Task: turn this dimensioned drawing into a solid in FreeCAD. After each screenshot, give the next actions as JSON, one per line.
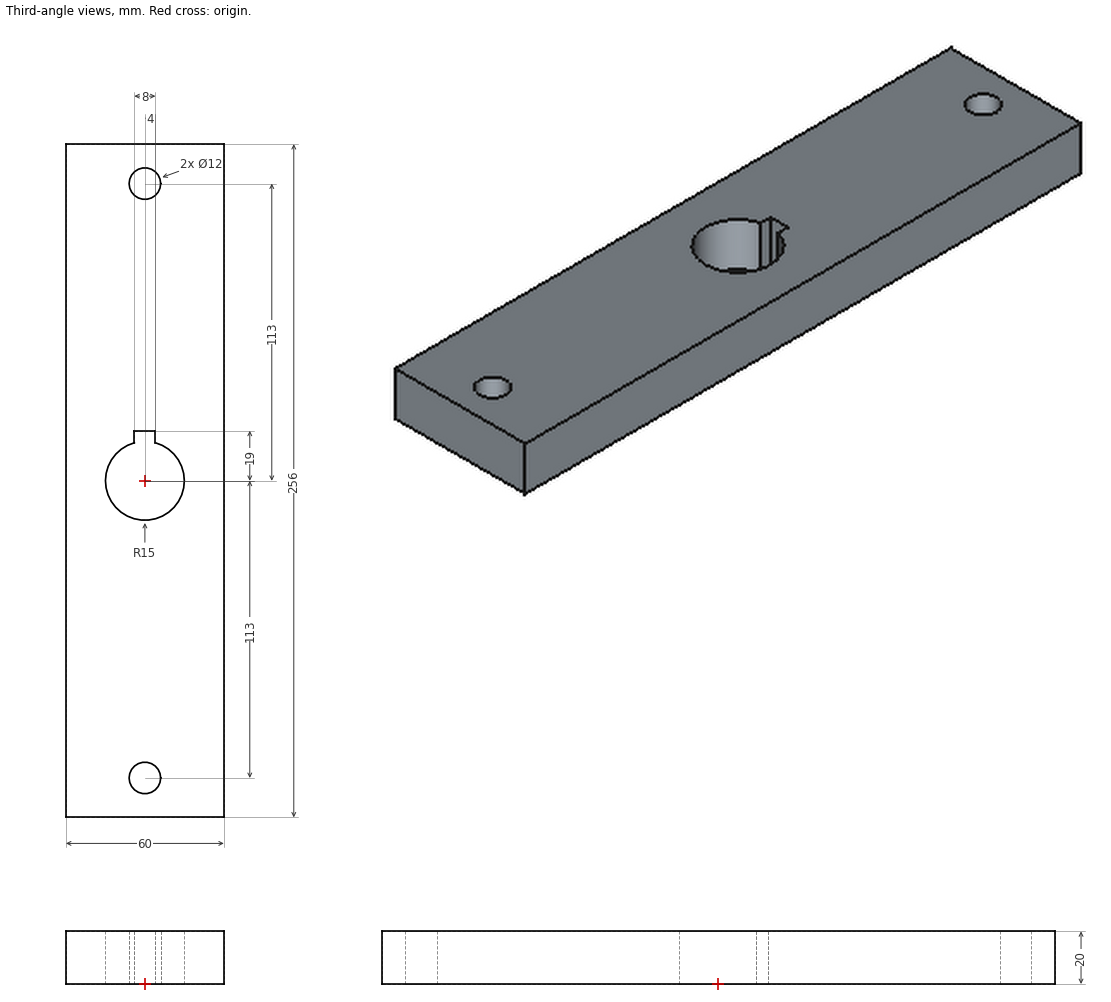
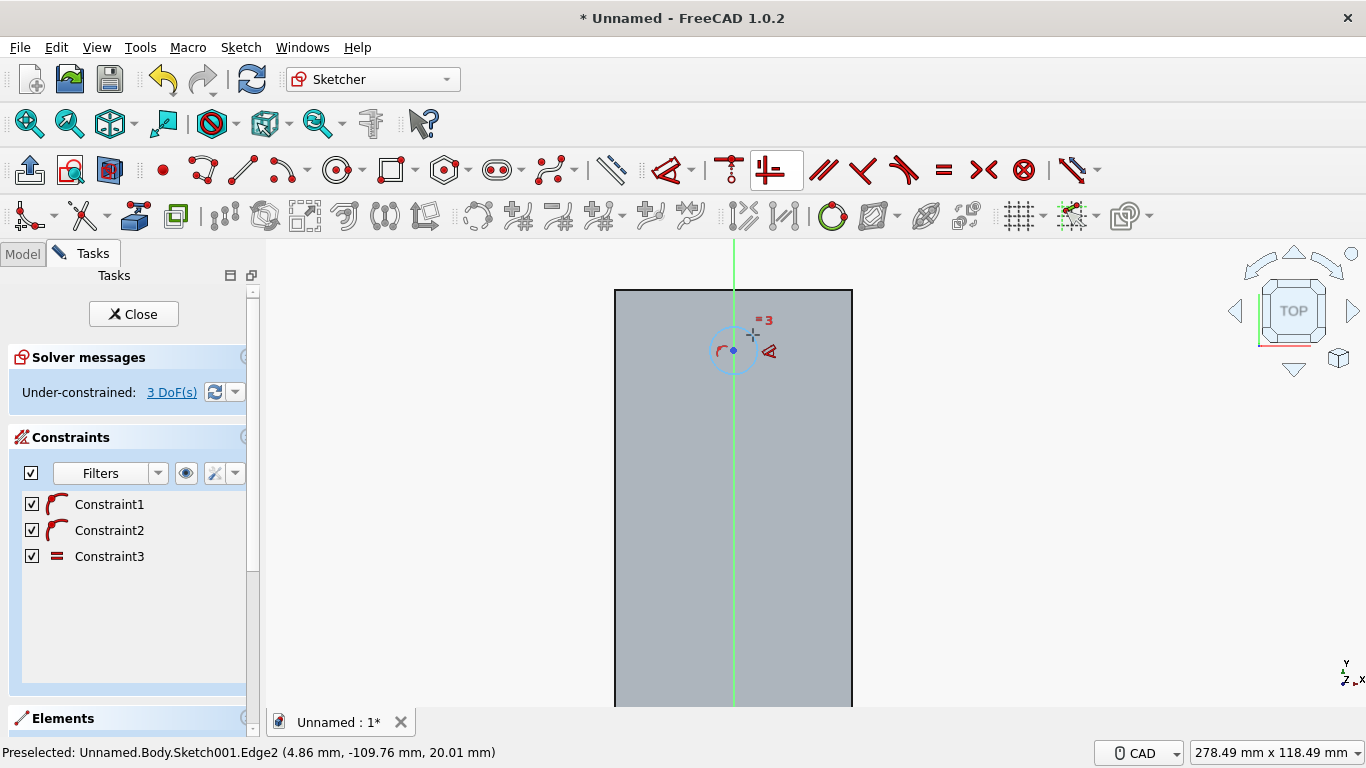
{"action": "left_click", "coordinate": [751, 334]}
{"action": "left_click", "coordinate": [774, 312]}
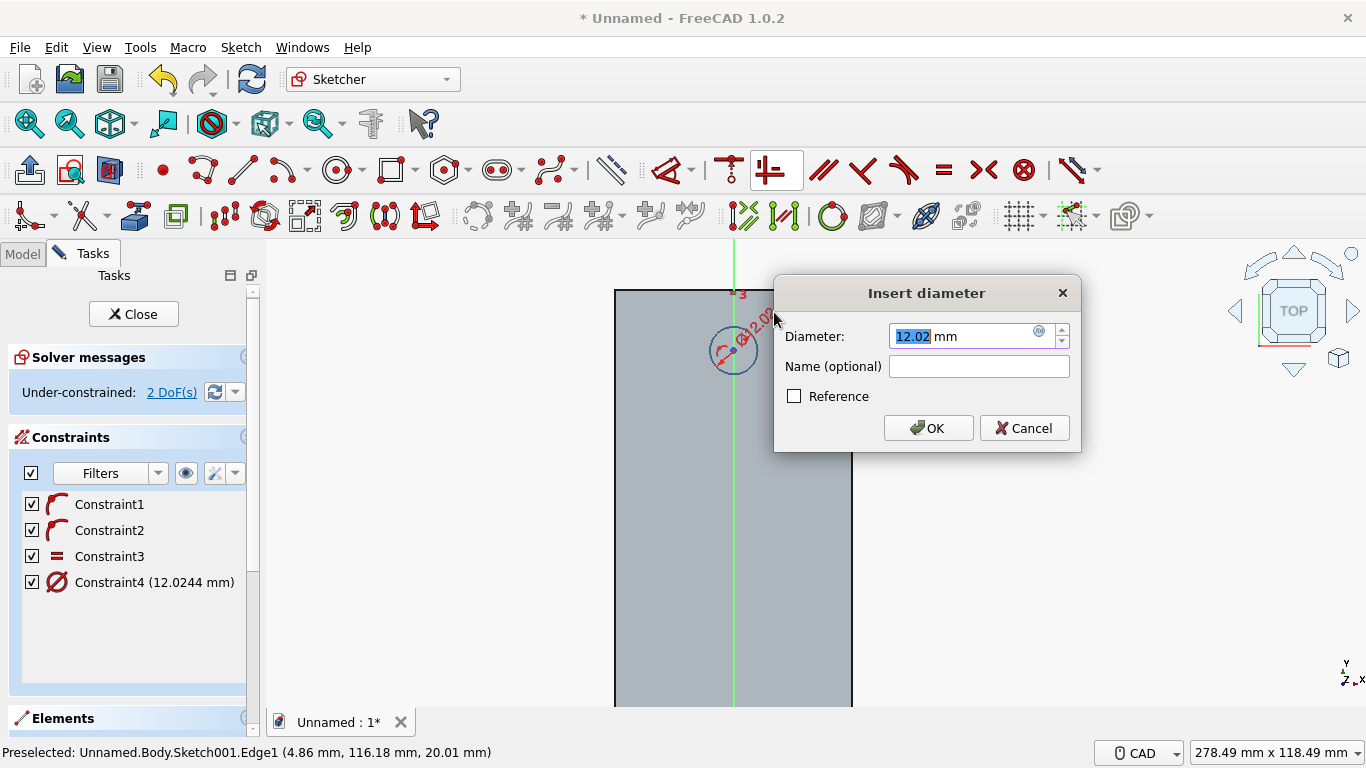
{"action": "type", "text": "12"}
{"action": "key", "text": "Return"}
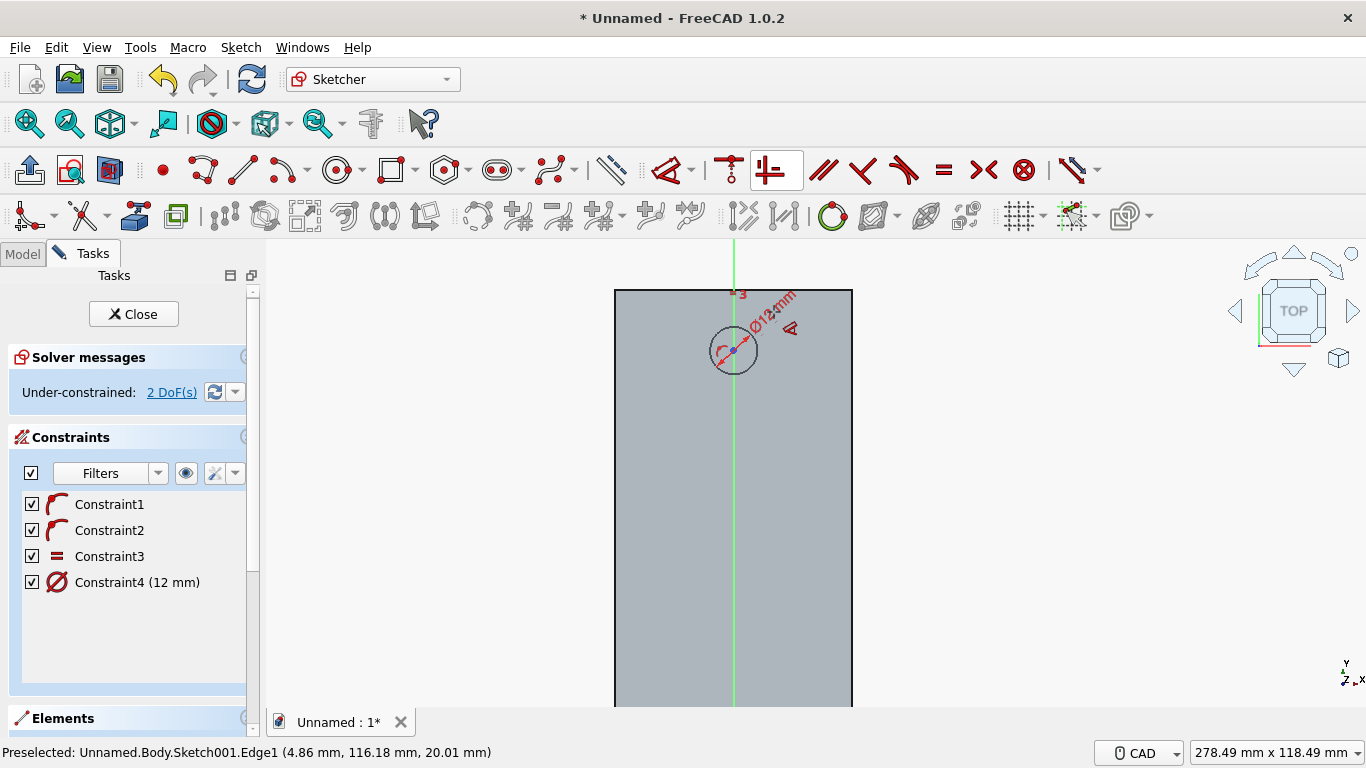
{"action": "left_click", "coordinate": [734, 351]}
{"action": "left_click", "coordinate": [768, 515]}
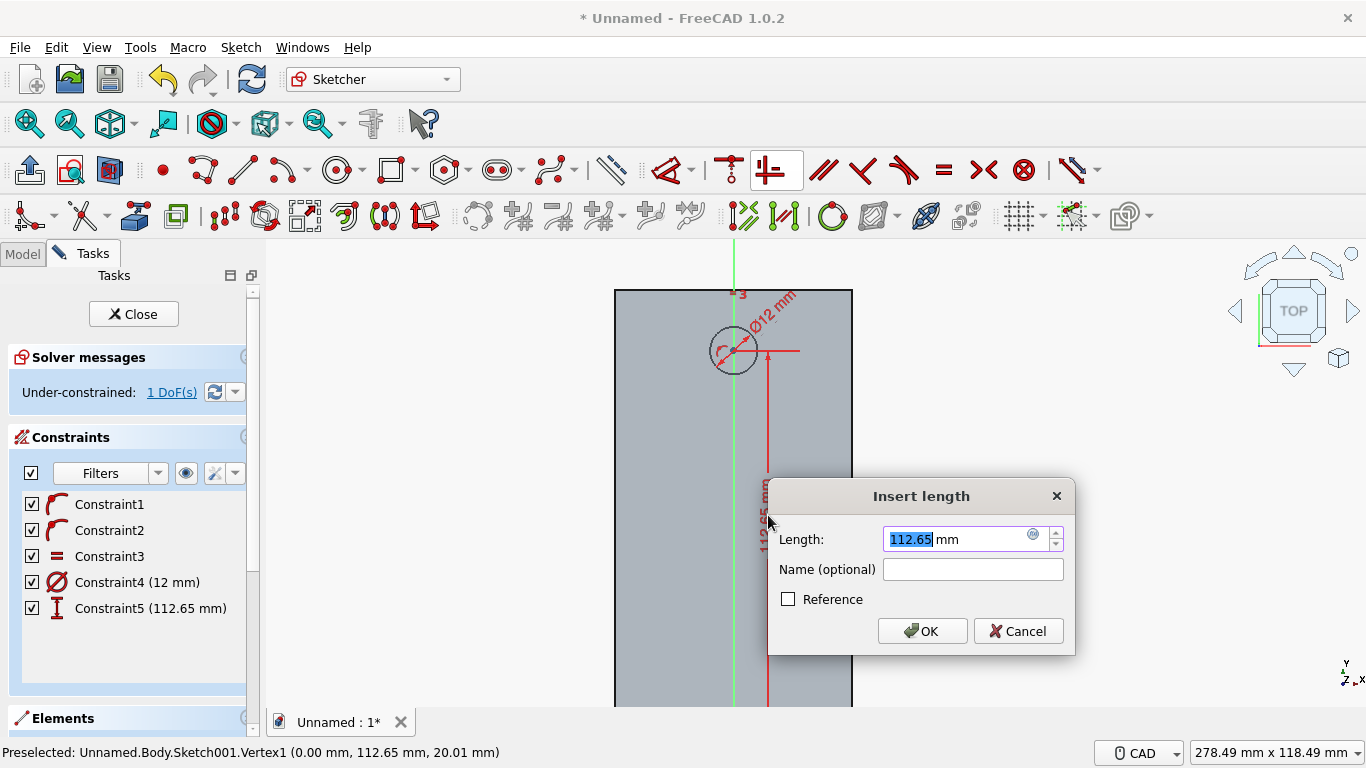
{"action": "type", "text": "113"}
{"action": "key", "text": "Return"}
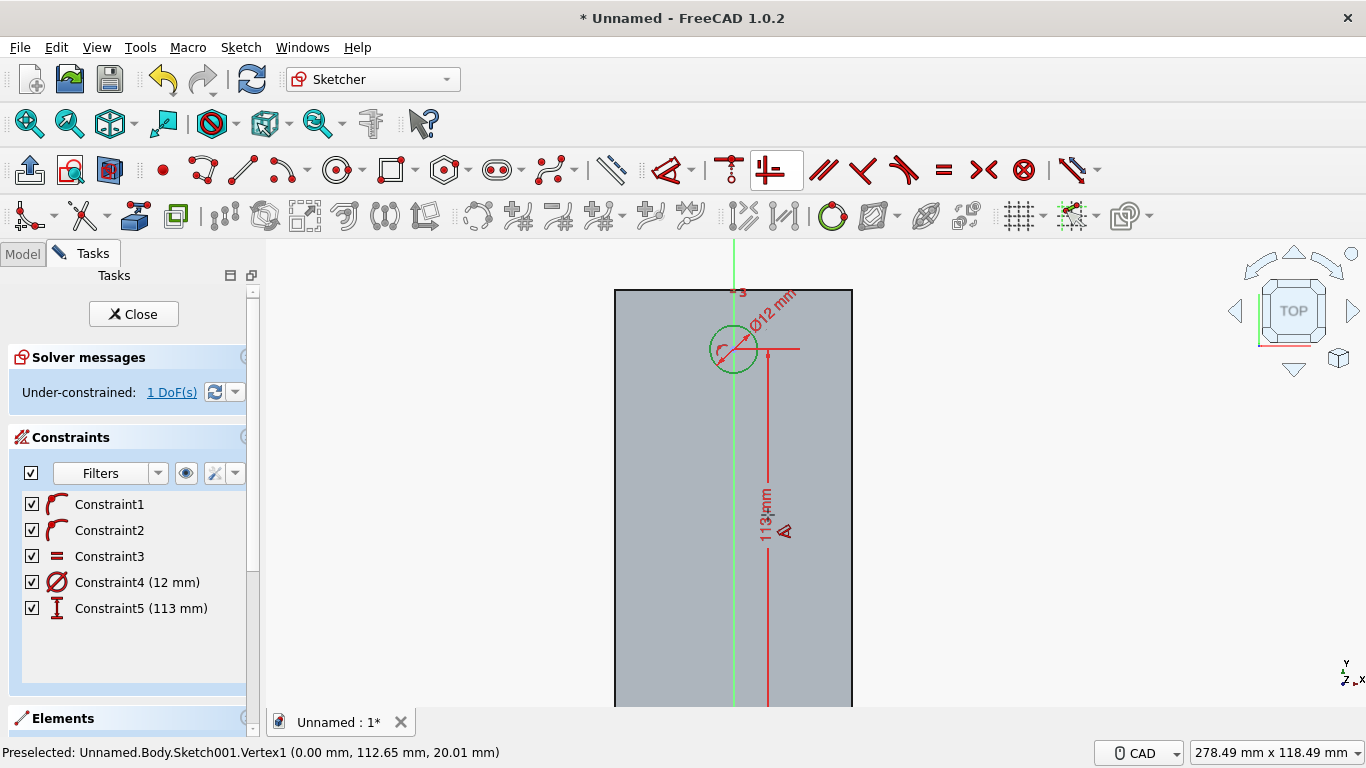
{"action": "scroll", "coordinate": [753, 334], "scroll_direction": "down", "scroll_amount": 6}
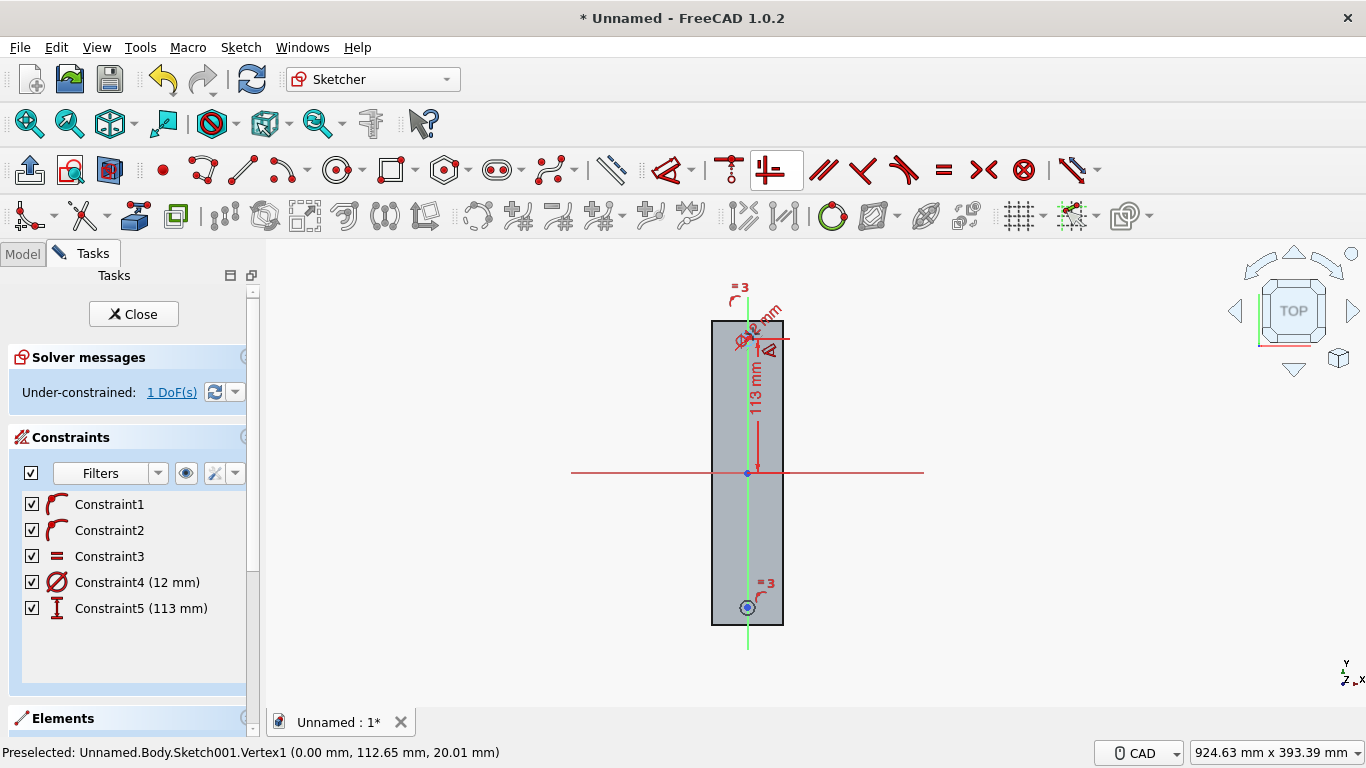
{"action": "left_click", "coordinate": [748, 608]}
{"action": "left_click", "coordinate": [782, 541]}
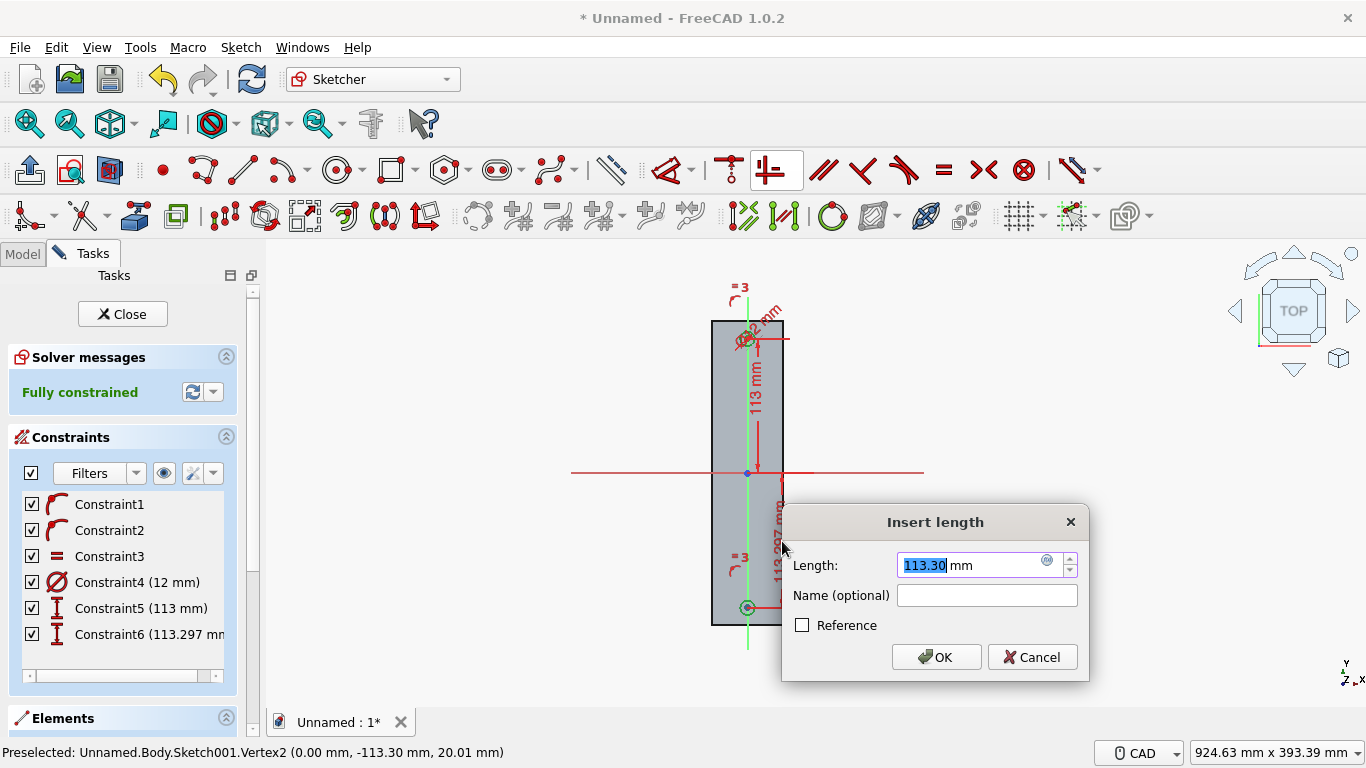
{"action": "type", "text": "113"}
{"action": "key", "text": "Return"}
{"action": "key", "text": "Escape"}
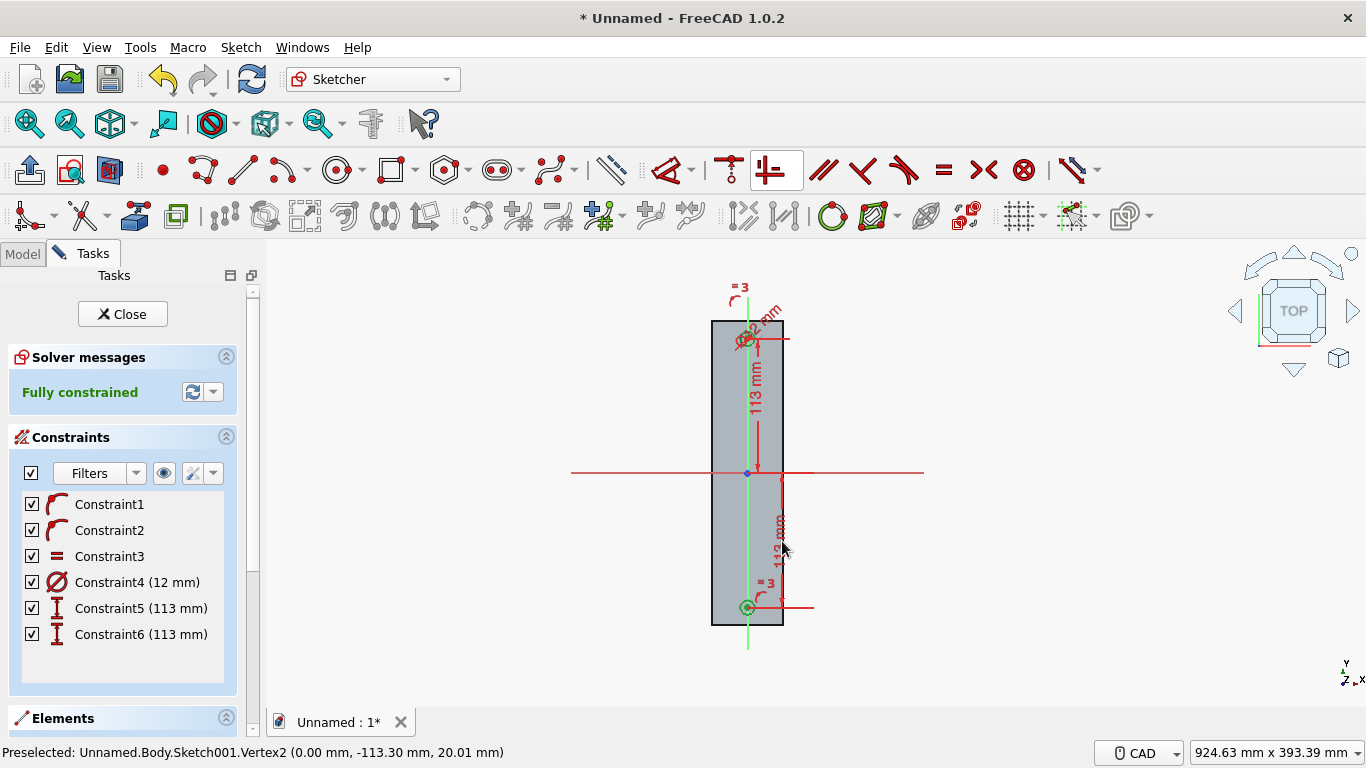
{"action": "left_click", "coordinate": [123, 314]}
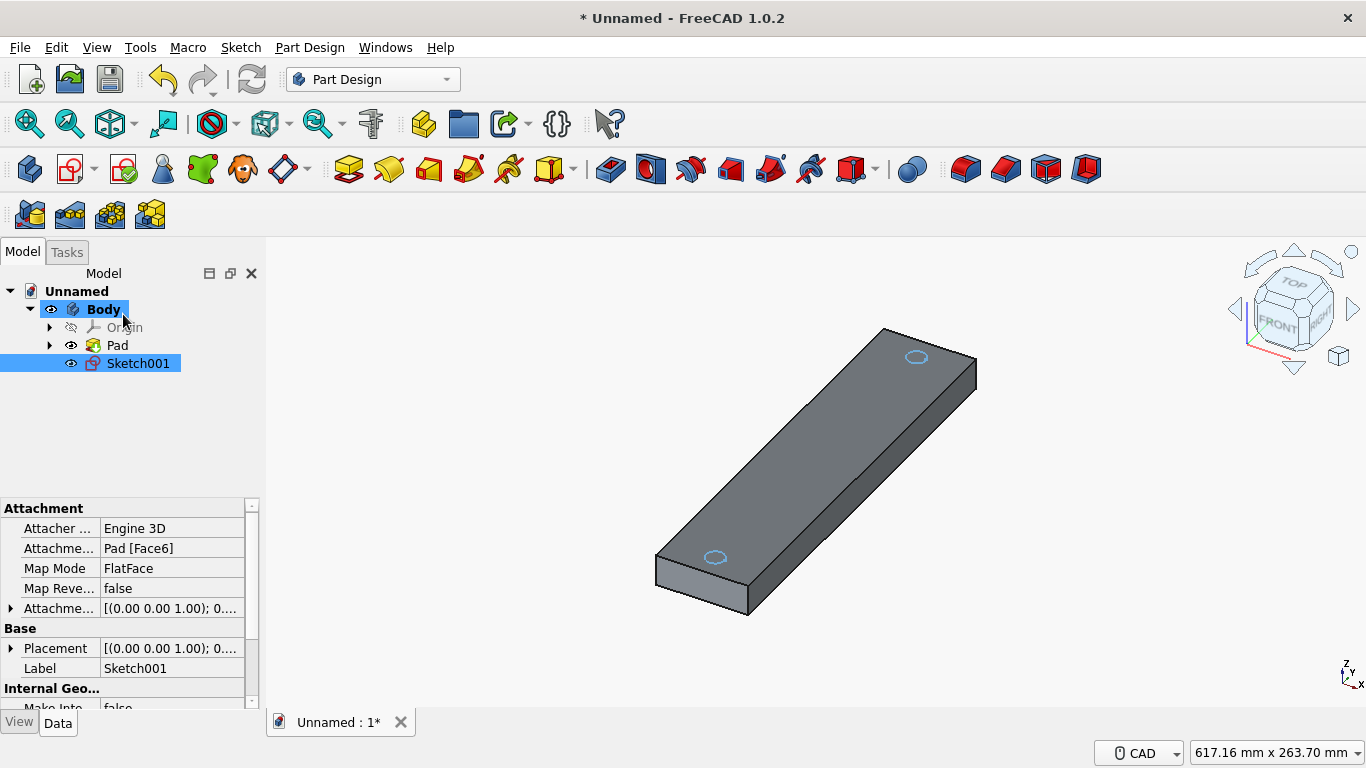
{"action": "left_click", "coordinate": [612, 170]}